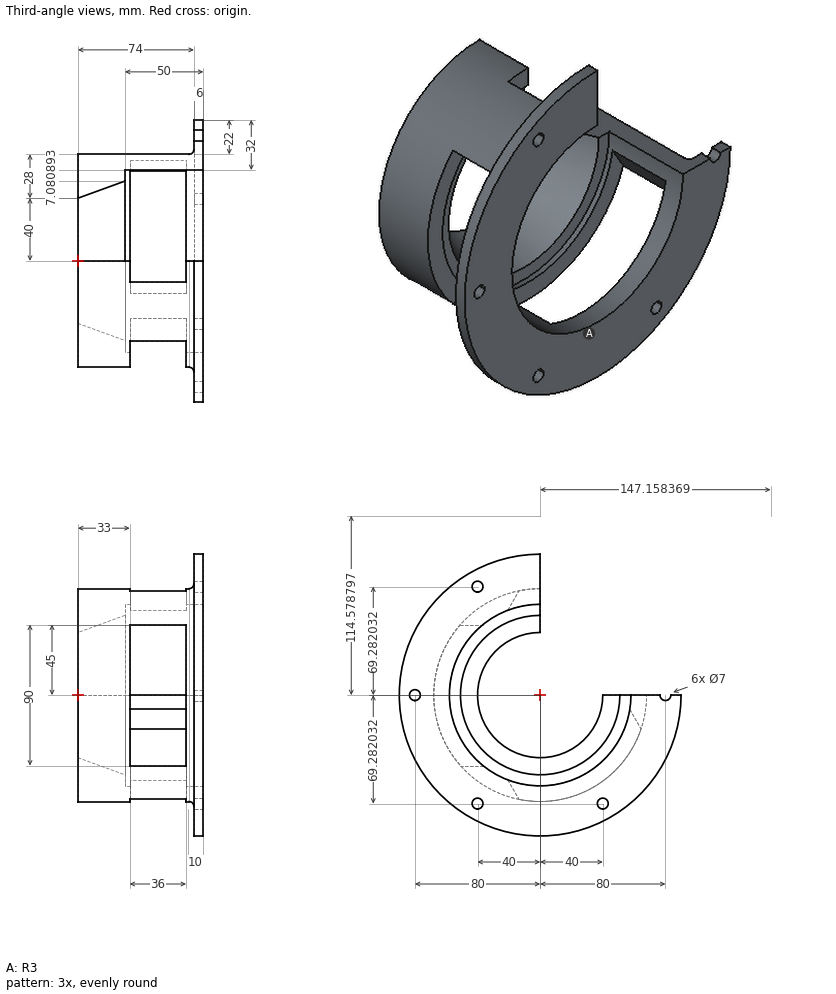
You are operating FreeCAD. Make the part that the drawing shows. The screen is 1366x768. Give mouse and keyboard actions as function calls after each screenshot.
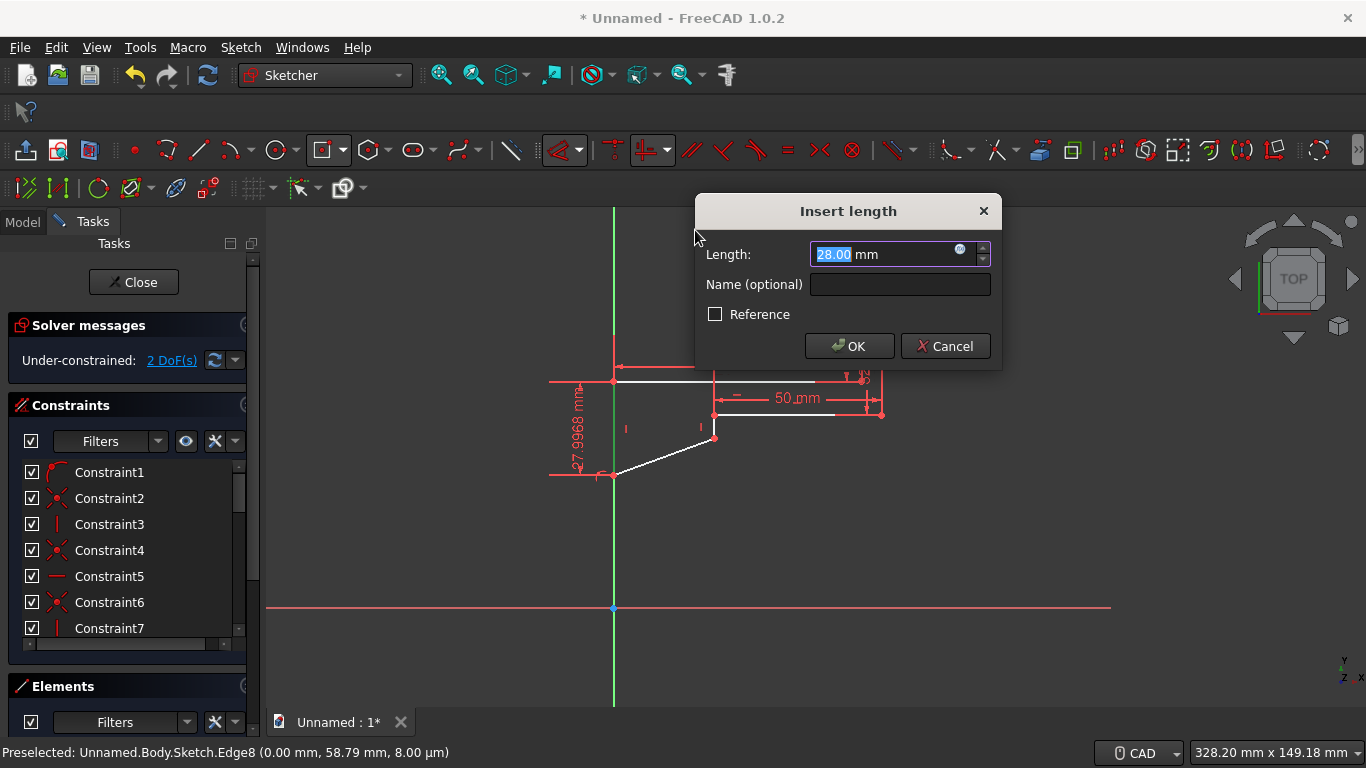
text(28)
key(Return)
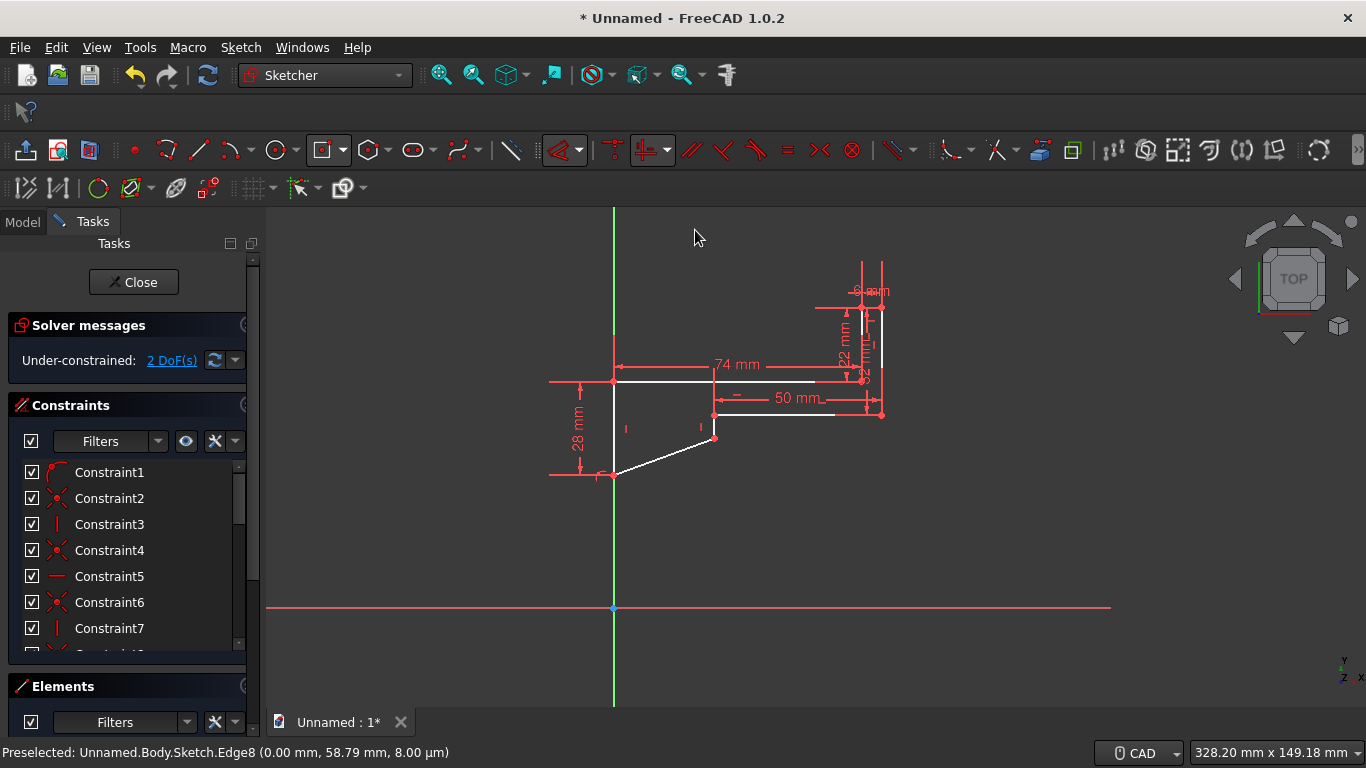
click(614, 475)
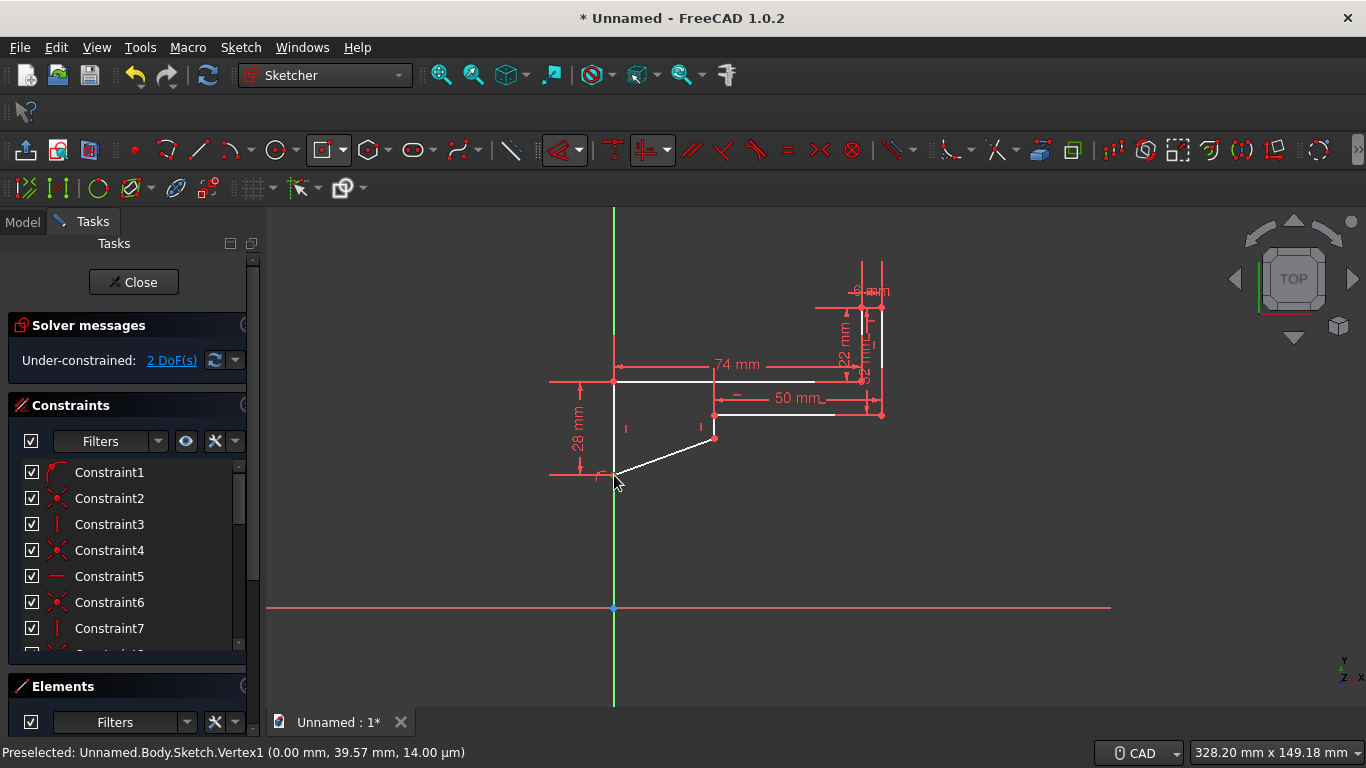
key(i)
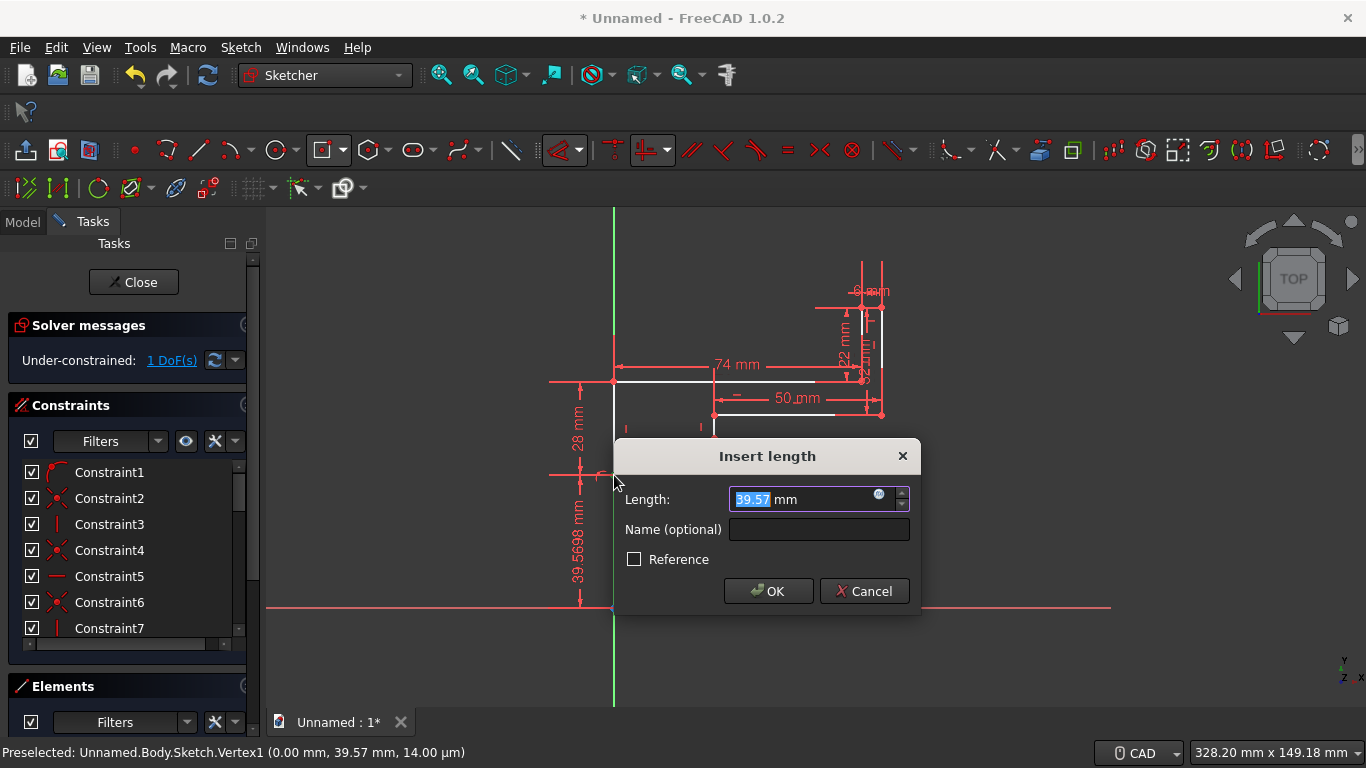
text(40)
key(Return)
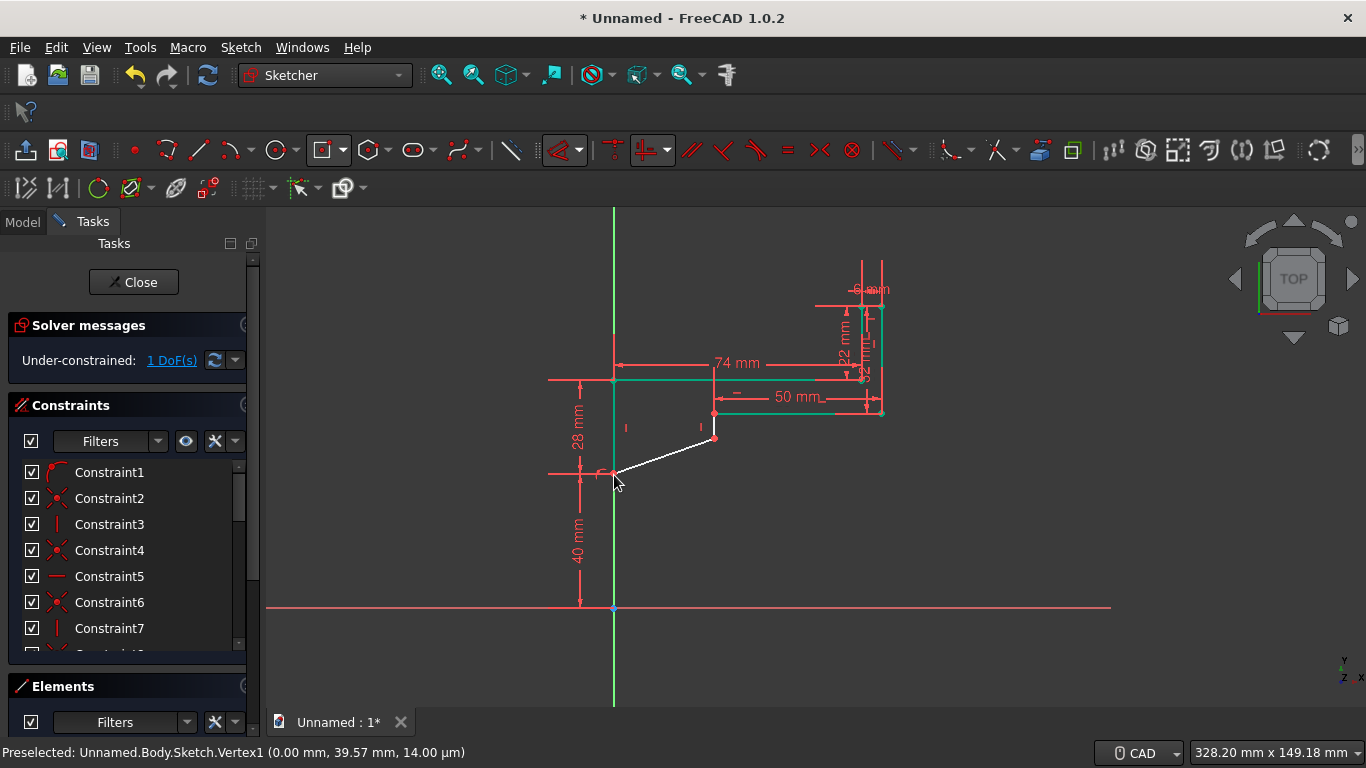
scroll(714, 429, up, 3)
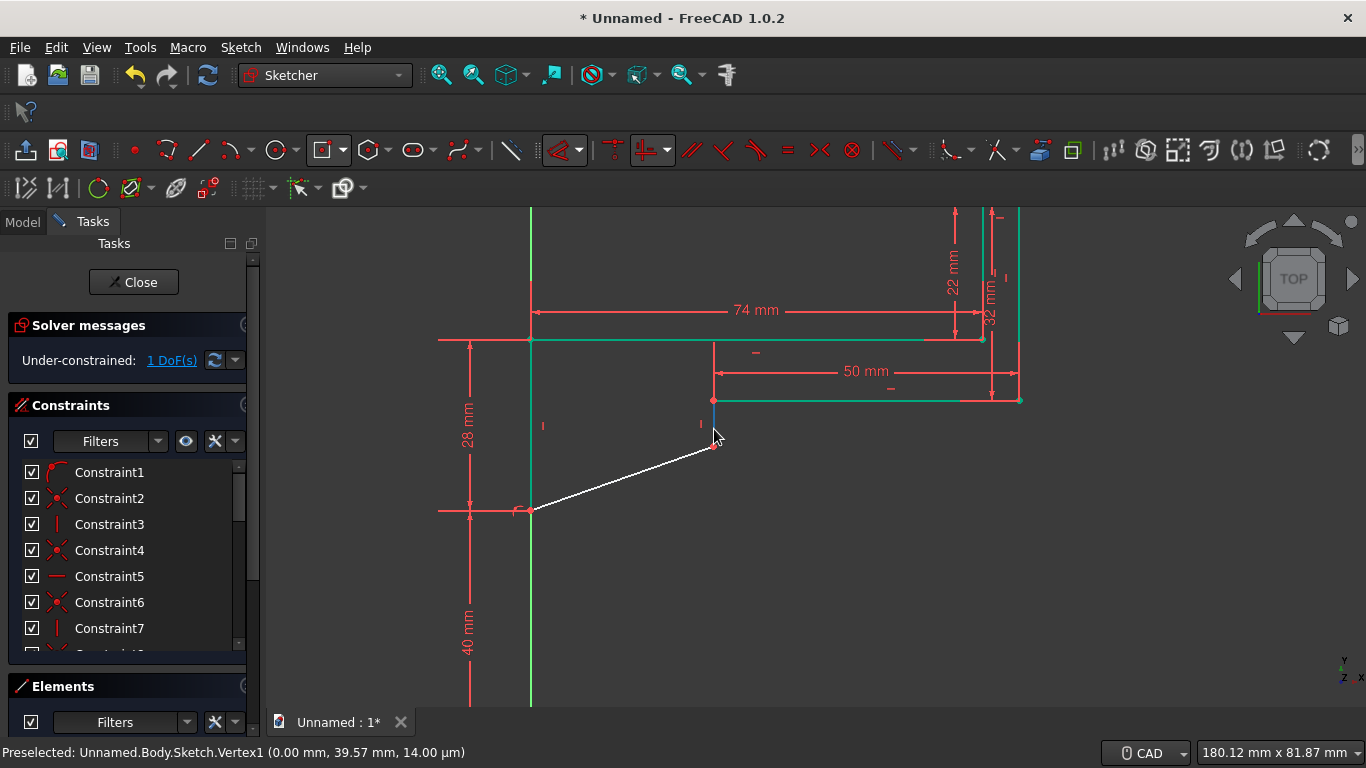
click(714, 428)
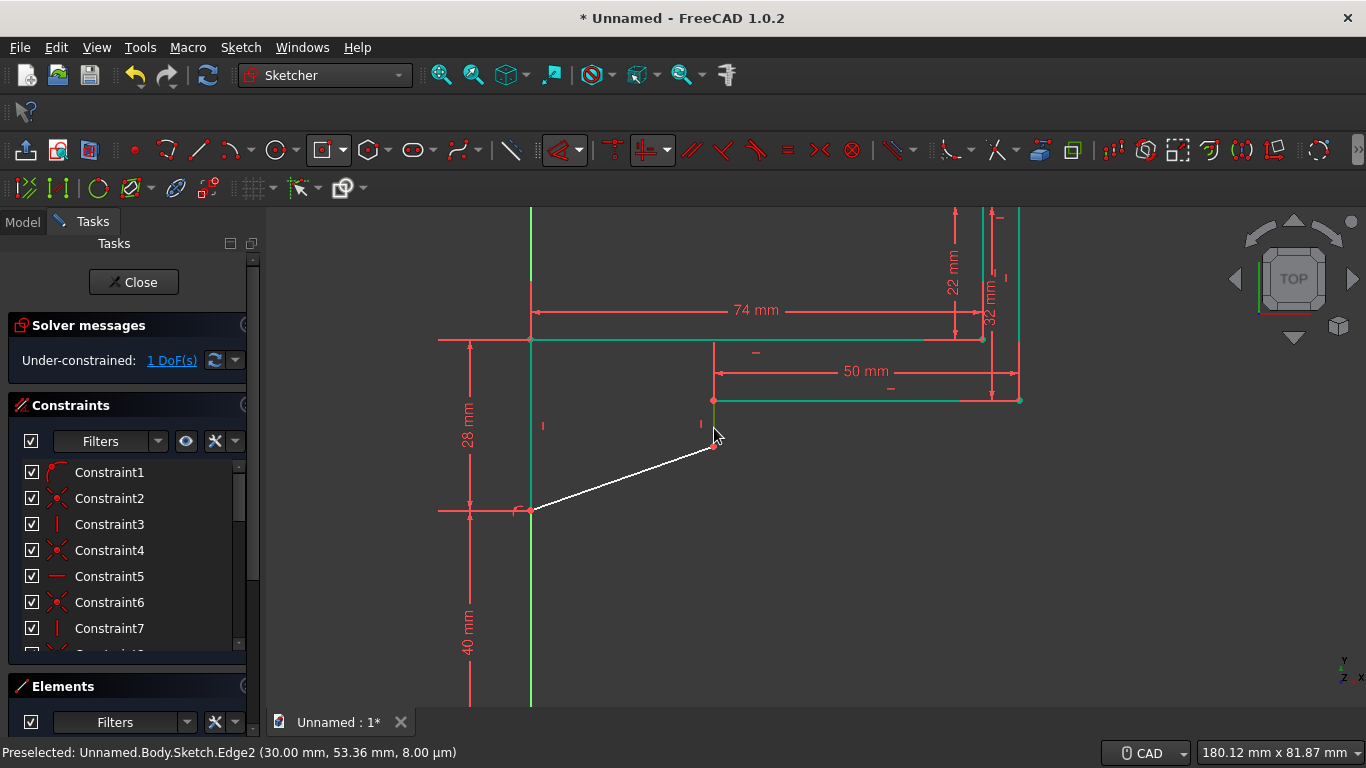
key(i)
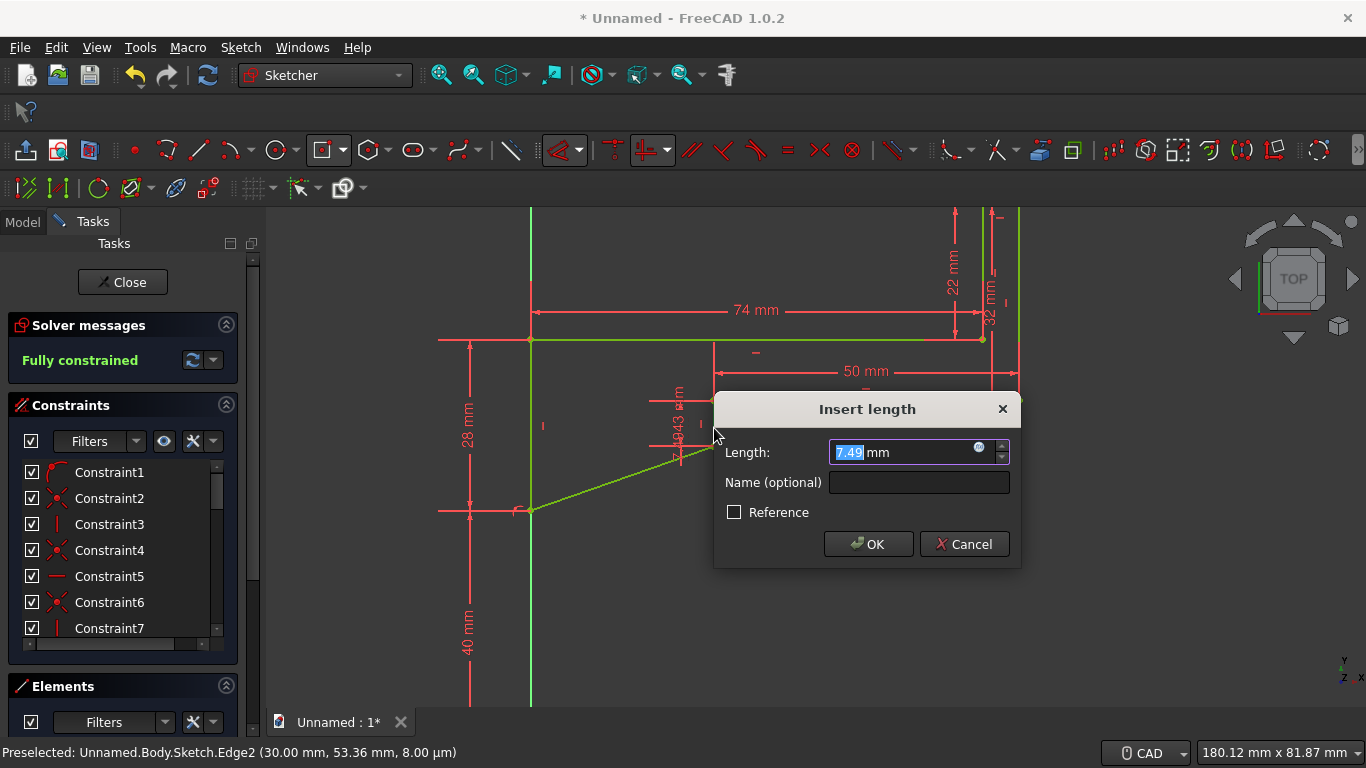
text(7.080893)
key(Return)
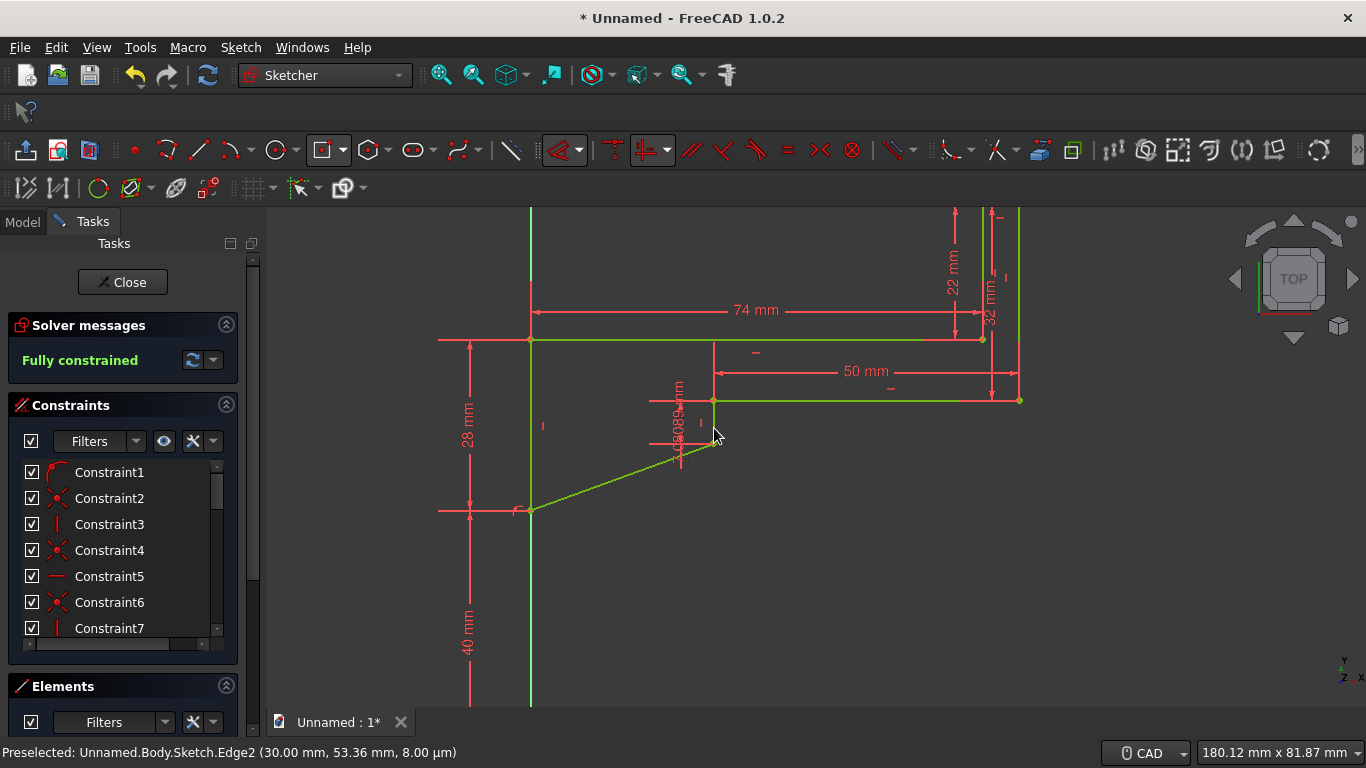
click(123, 282)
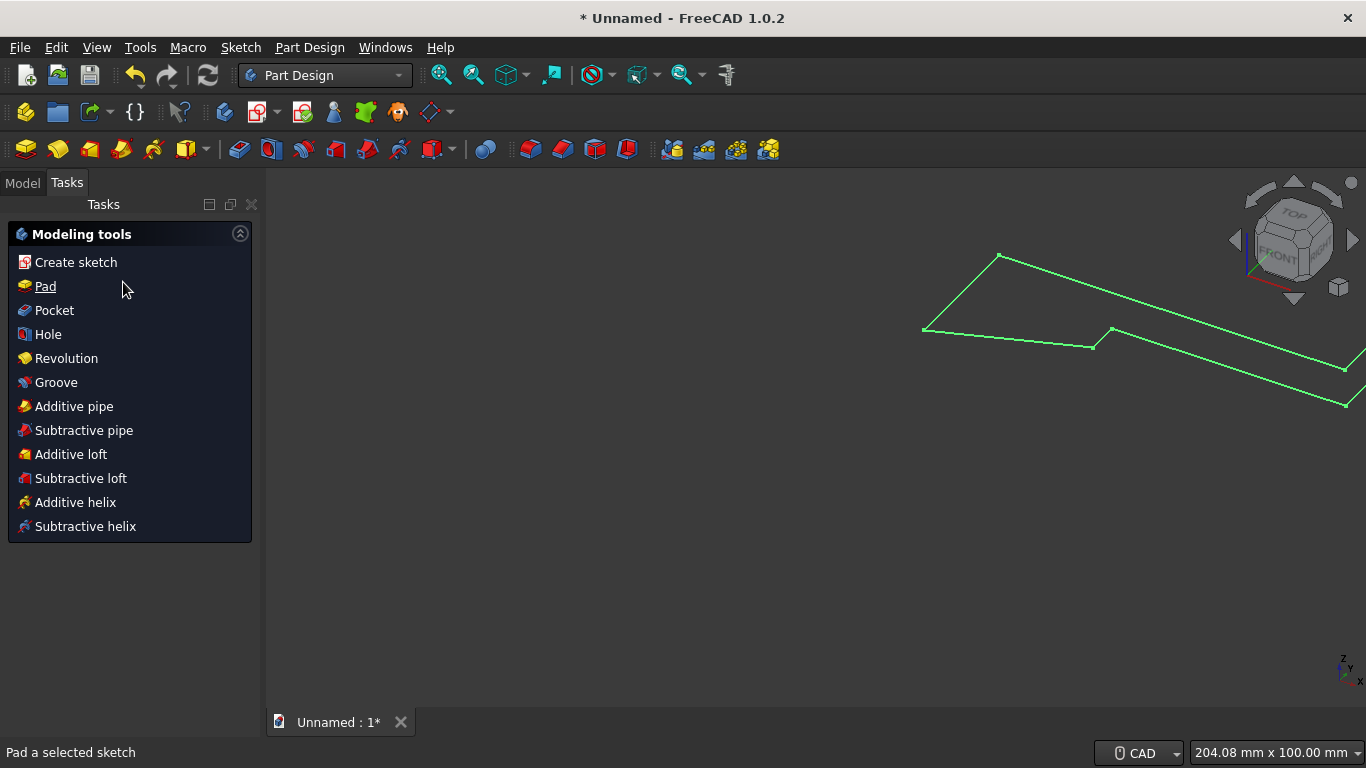
click(58, 150)